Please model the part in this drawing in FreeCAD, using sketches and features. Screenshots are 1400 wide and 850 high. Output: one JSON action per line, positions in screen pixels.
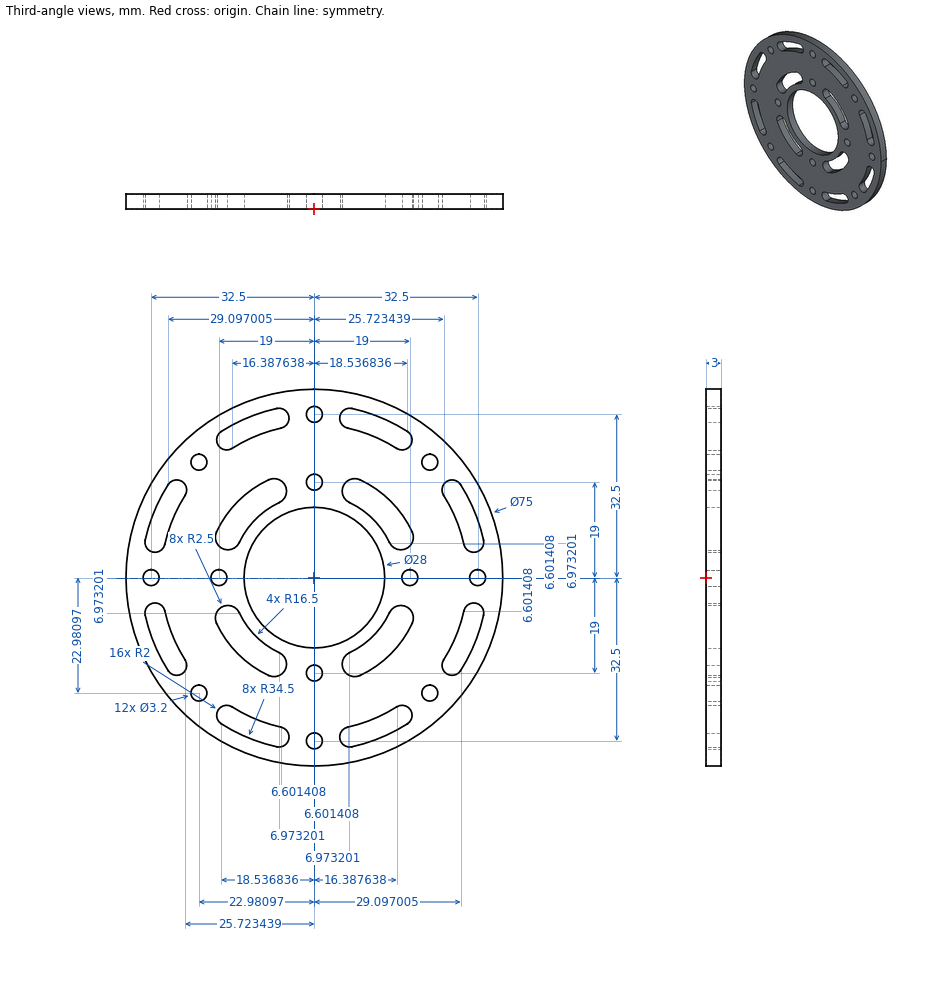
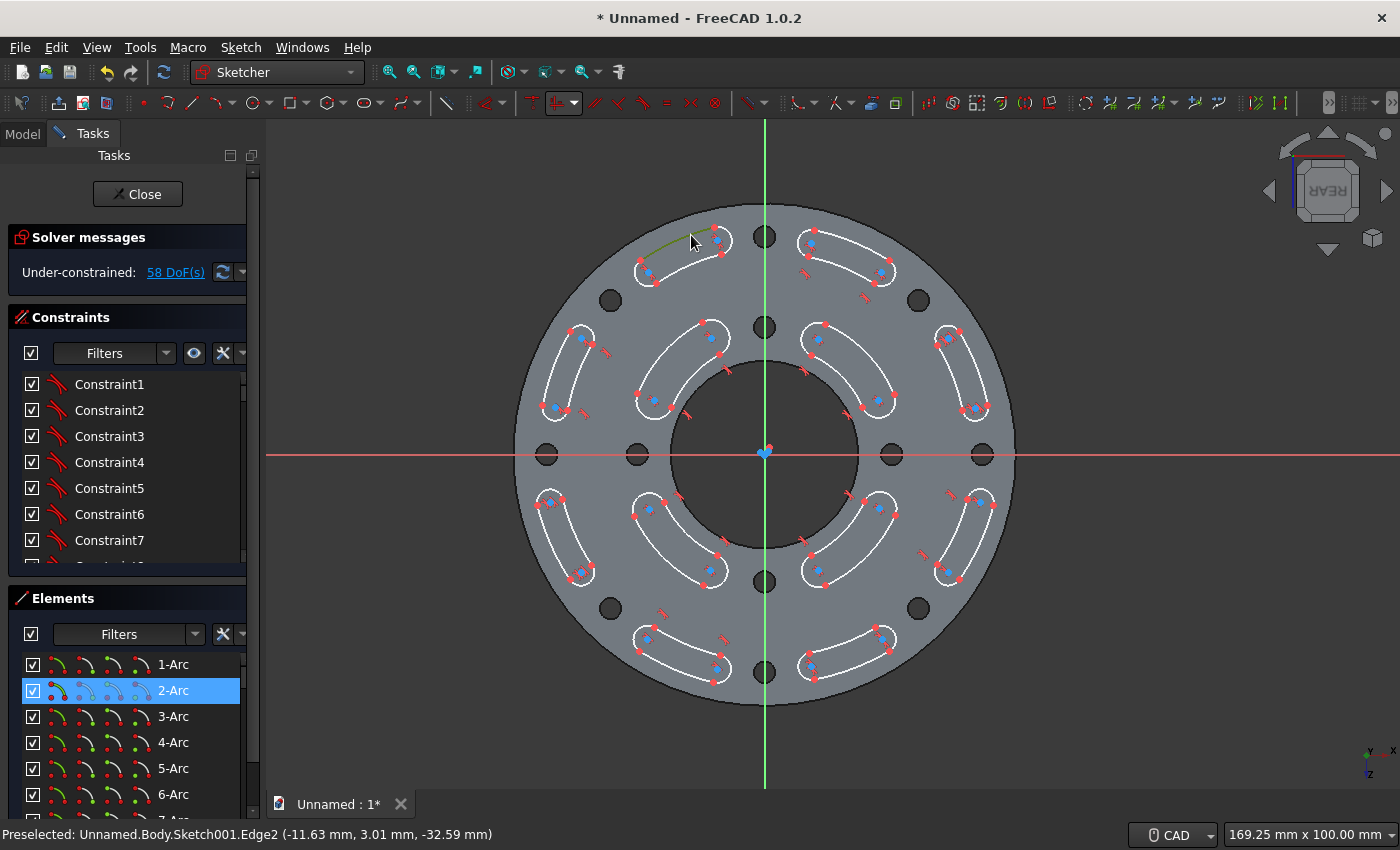
{"action": "left_click", "coordinate": [831, 543]}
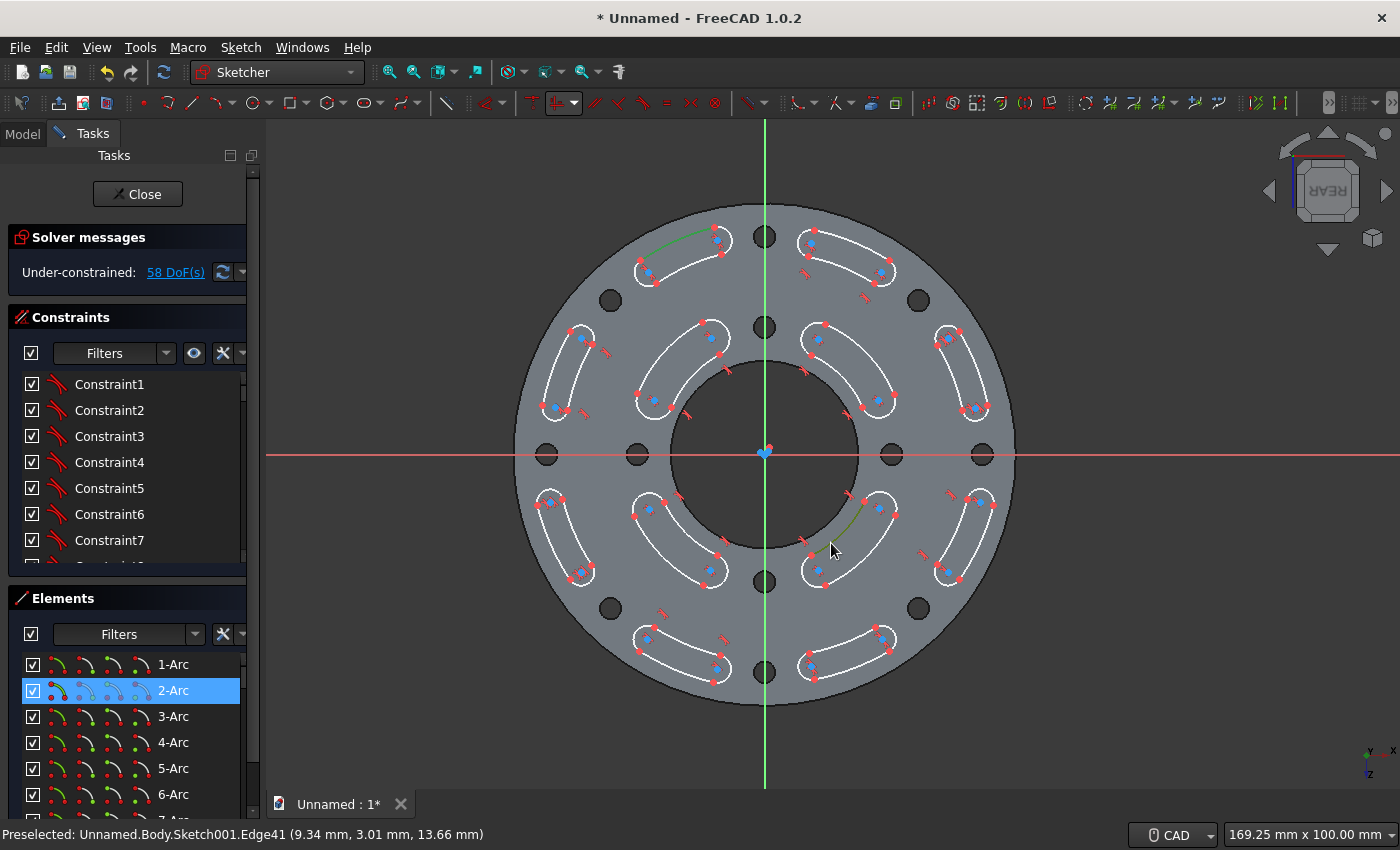
{"action": "left_click", "coordinate": [532, 104]}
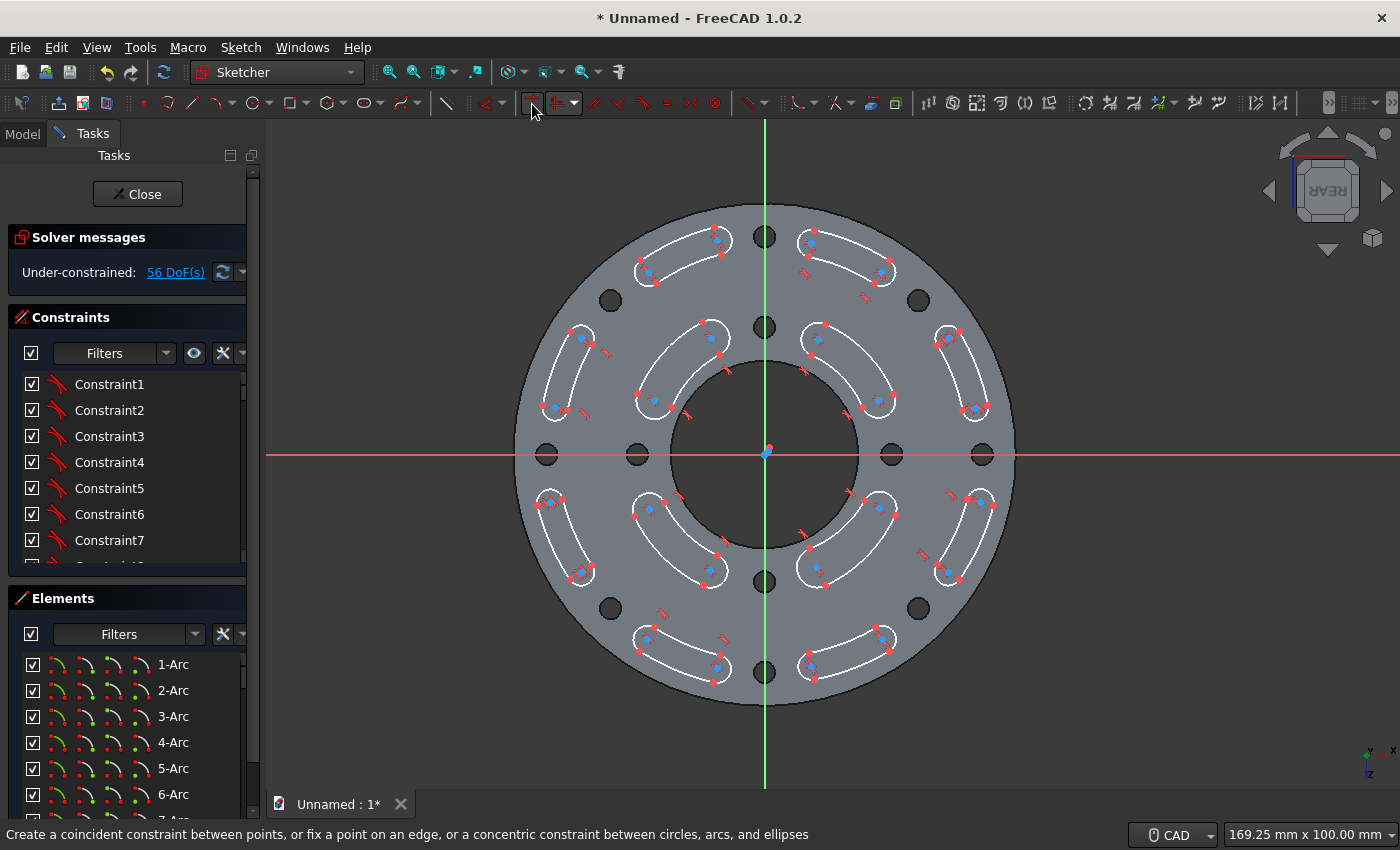
{"action": "left_click", "coordinate": [691, 235]}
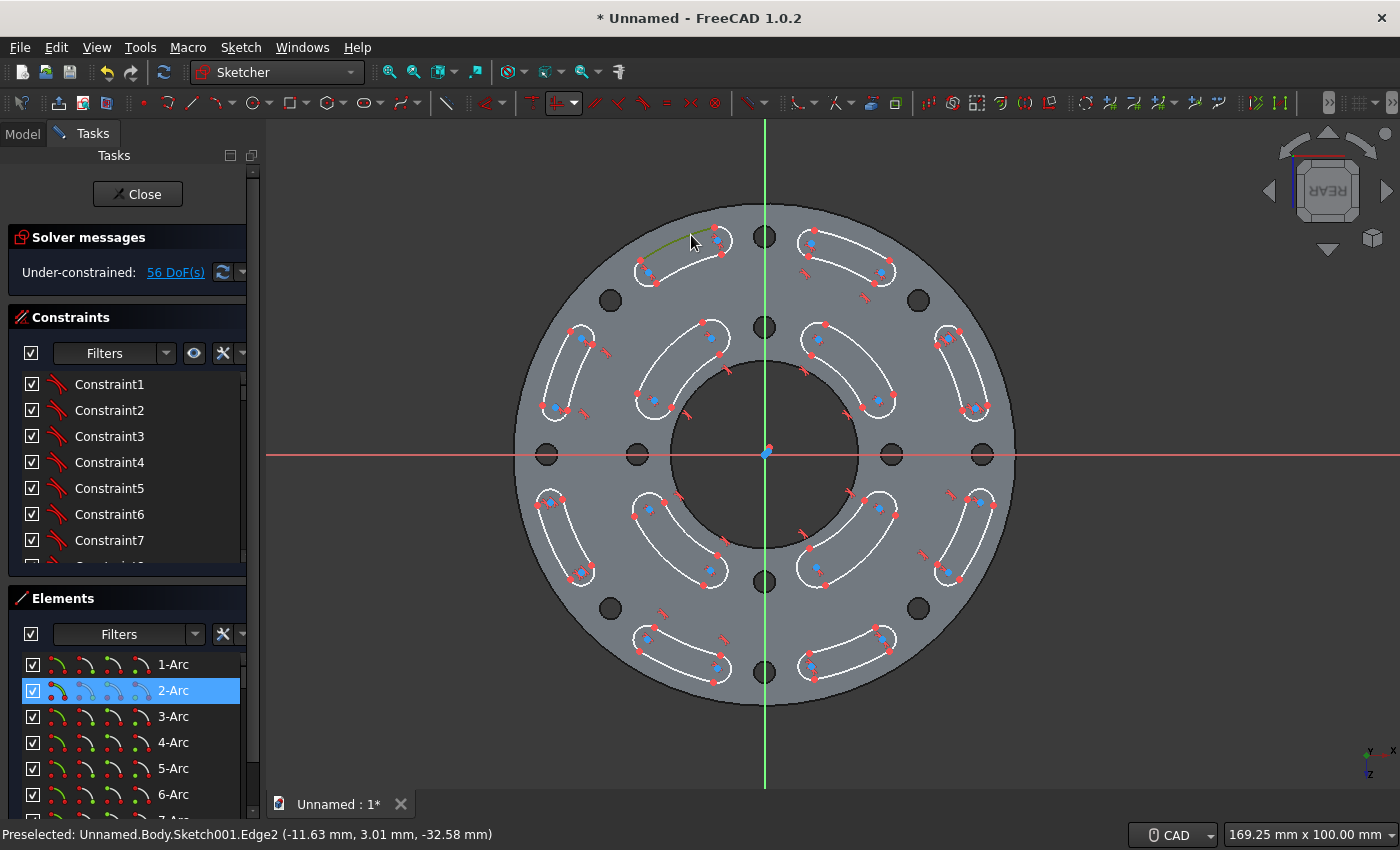
{"action": "left_click", "coordinate": [851, 570]}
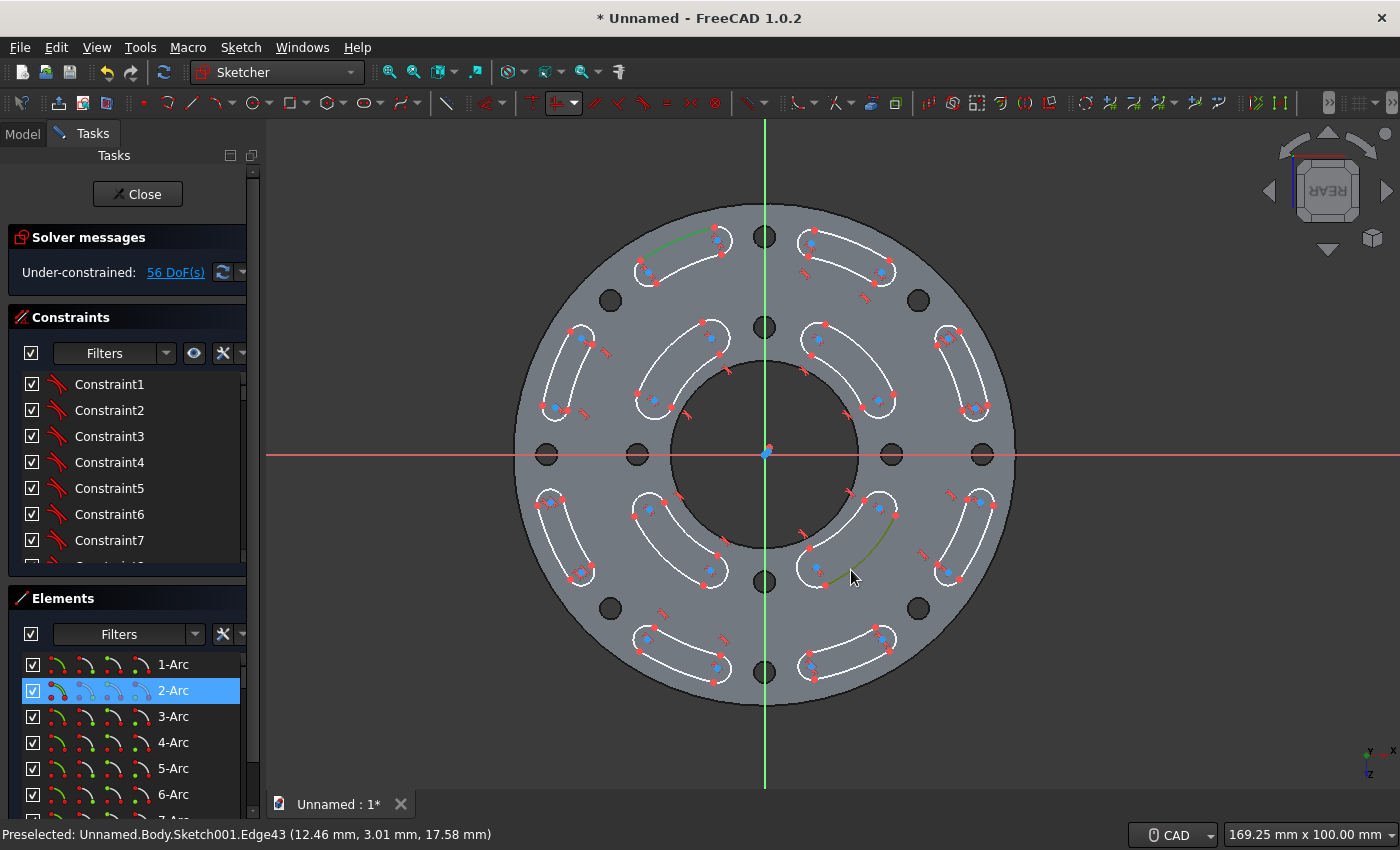
{"action": "left_click", "coordinate": [532, 104]}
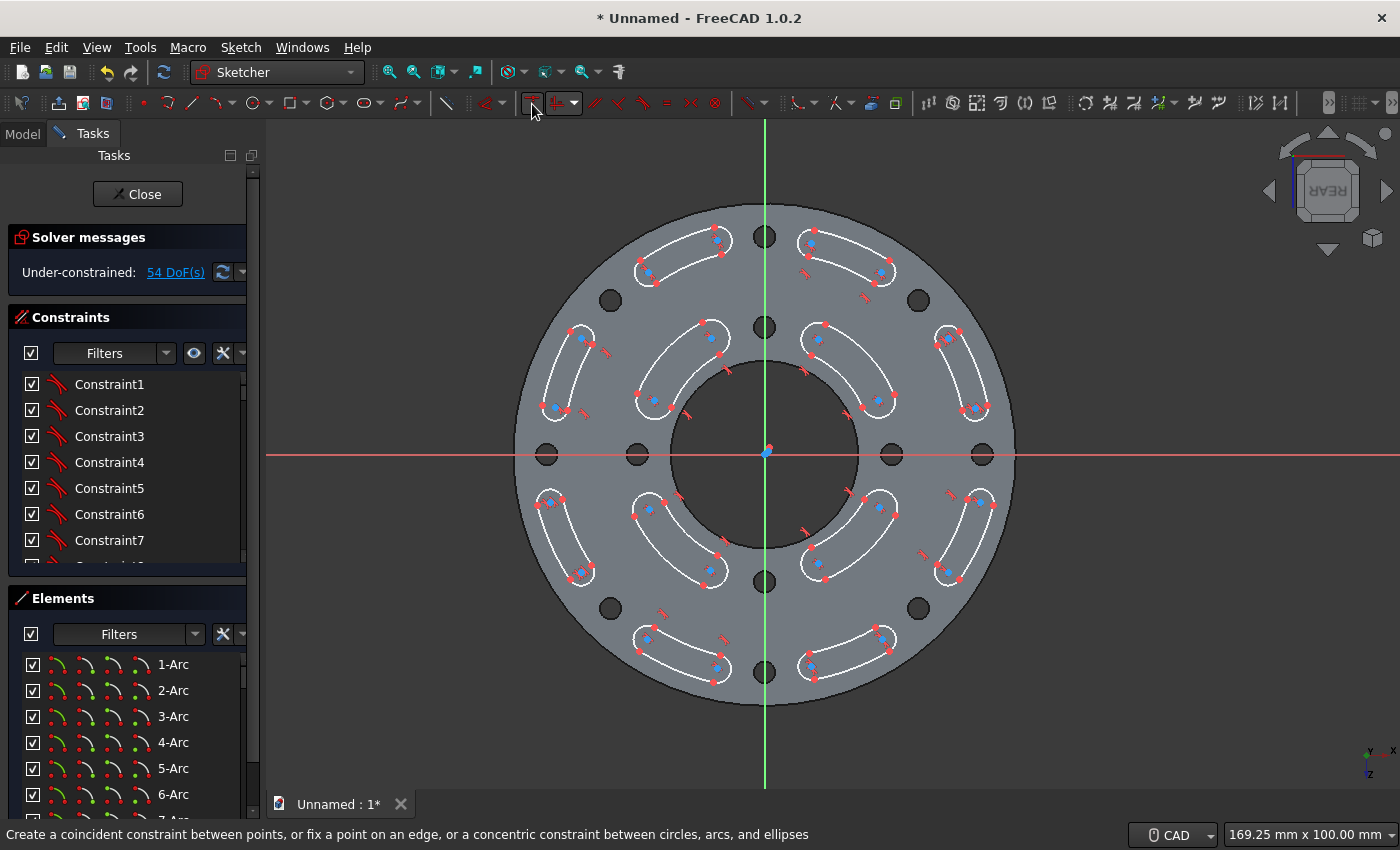
{"action": "left_click", "coordinate": [691, 235]}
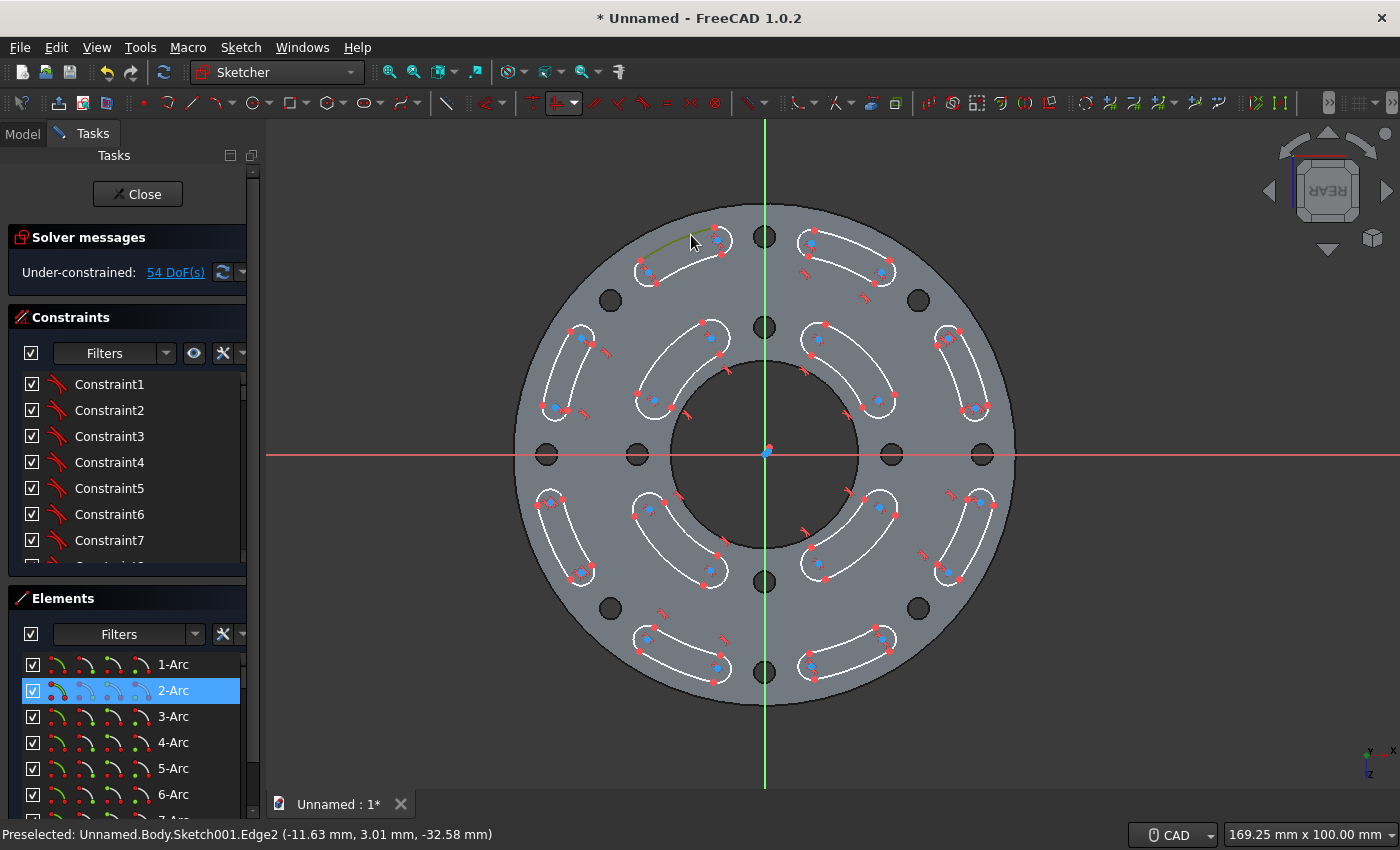
{"action": "left_click", "coordinate": [676, 522]}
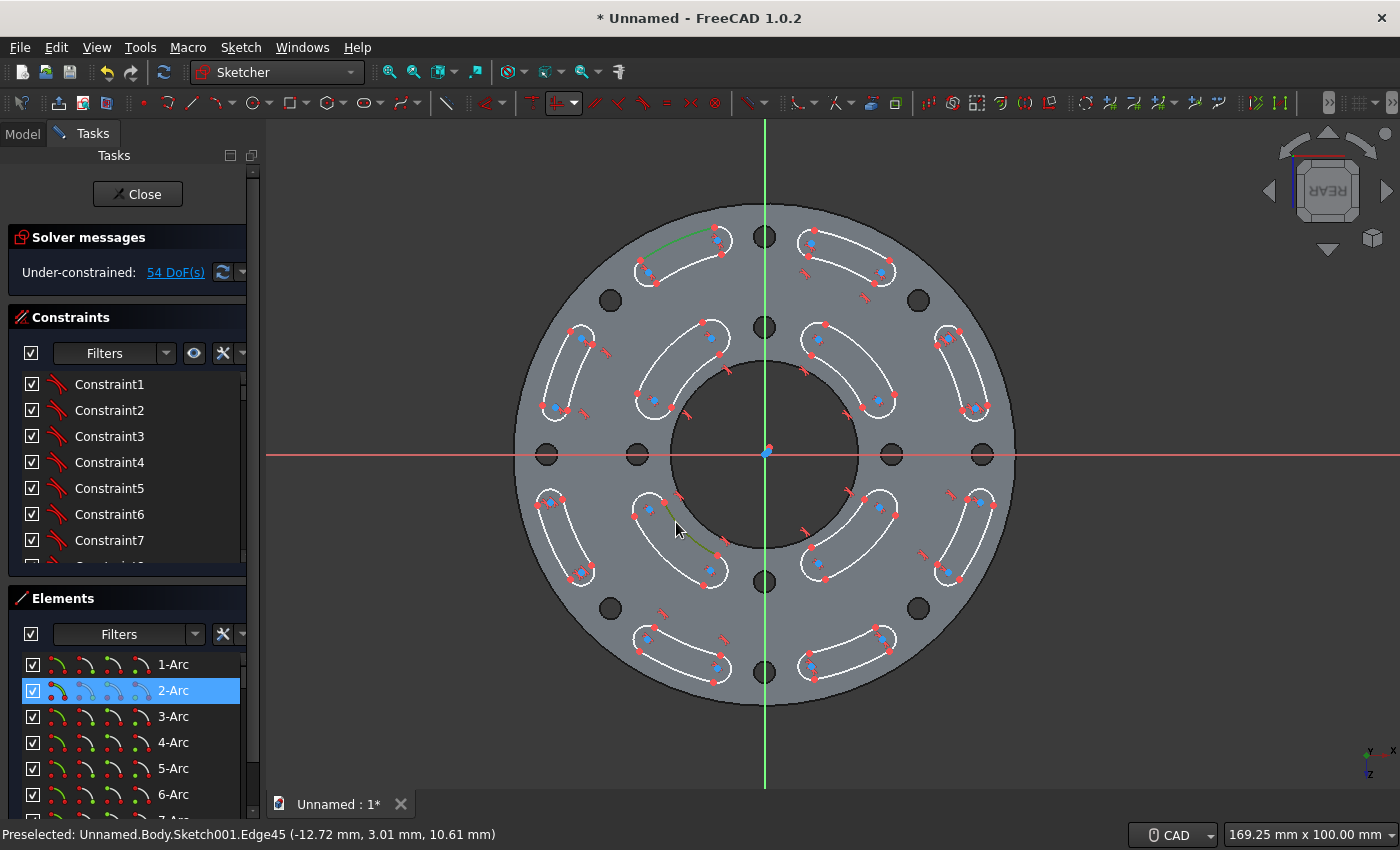
{"action": "left_click", "coordinate": [532, 104]}